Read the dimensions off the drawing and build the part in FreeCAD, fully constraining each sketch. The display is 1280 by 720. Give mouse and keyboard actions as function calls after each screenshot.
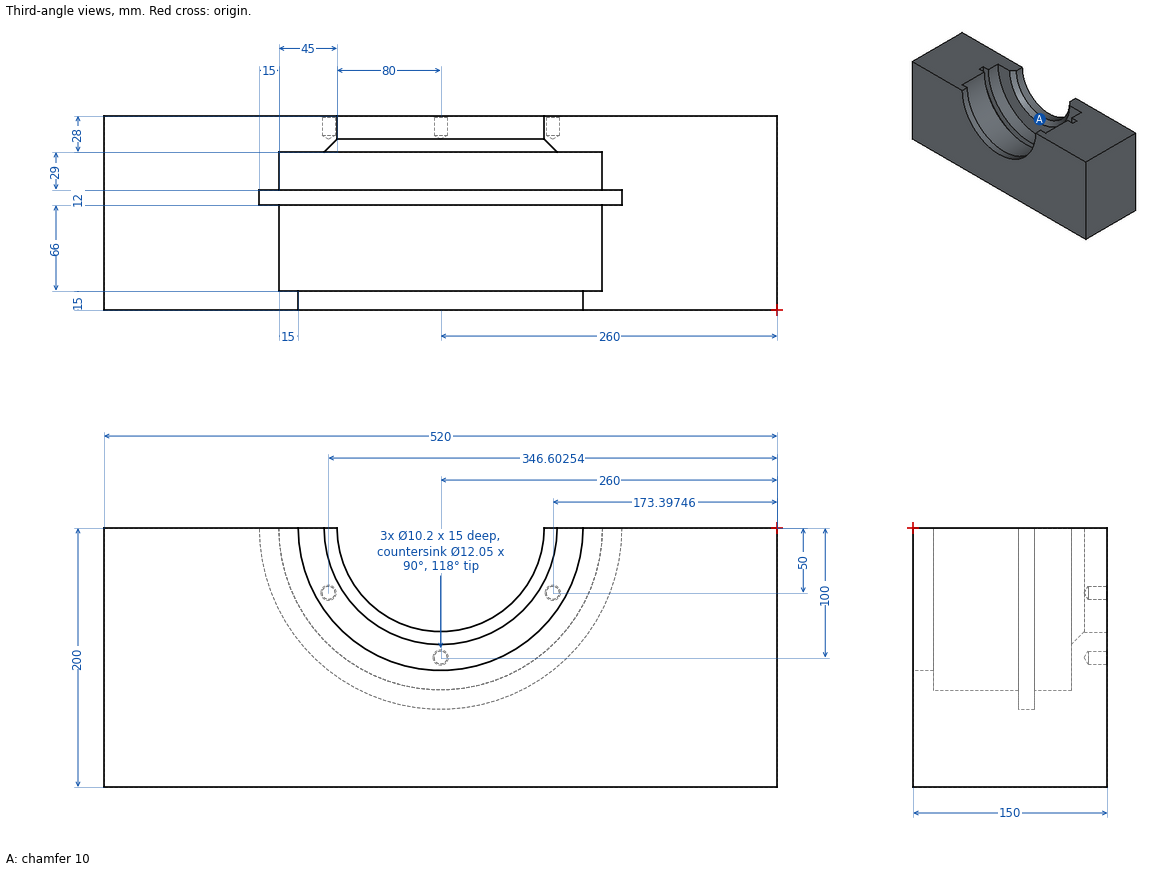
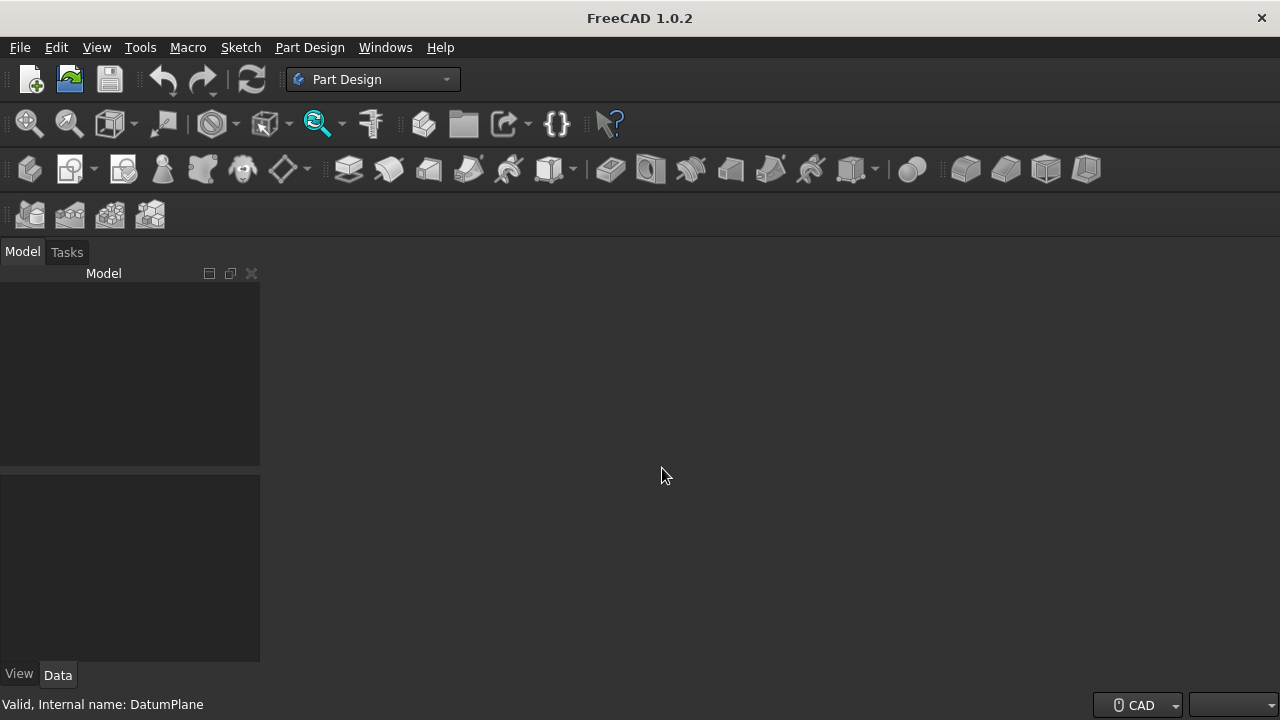
click(30, 80)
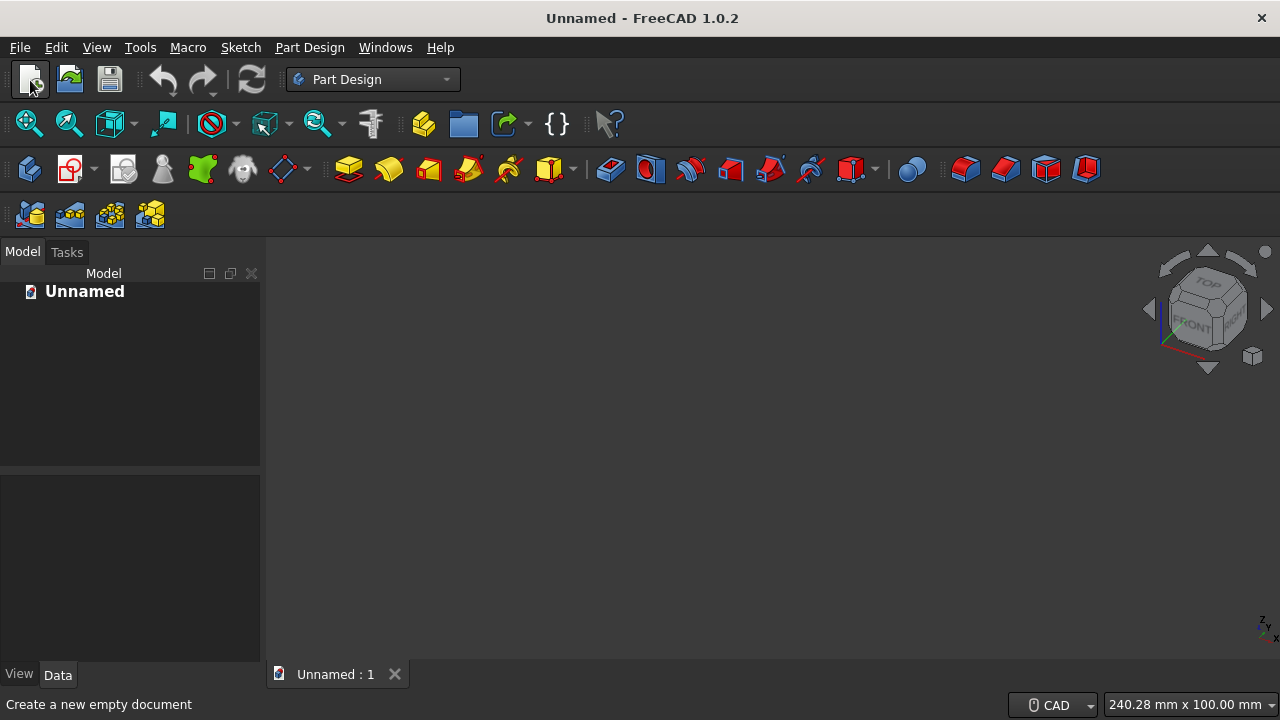
click(70, 170)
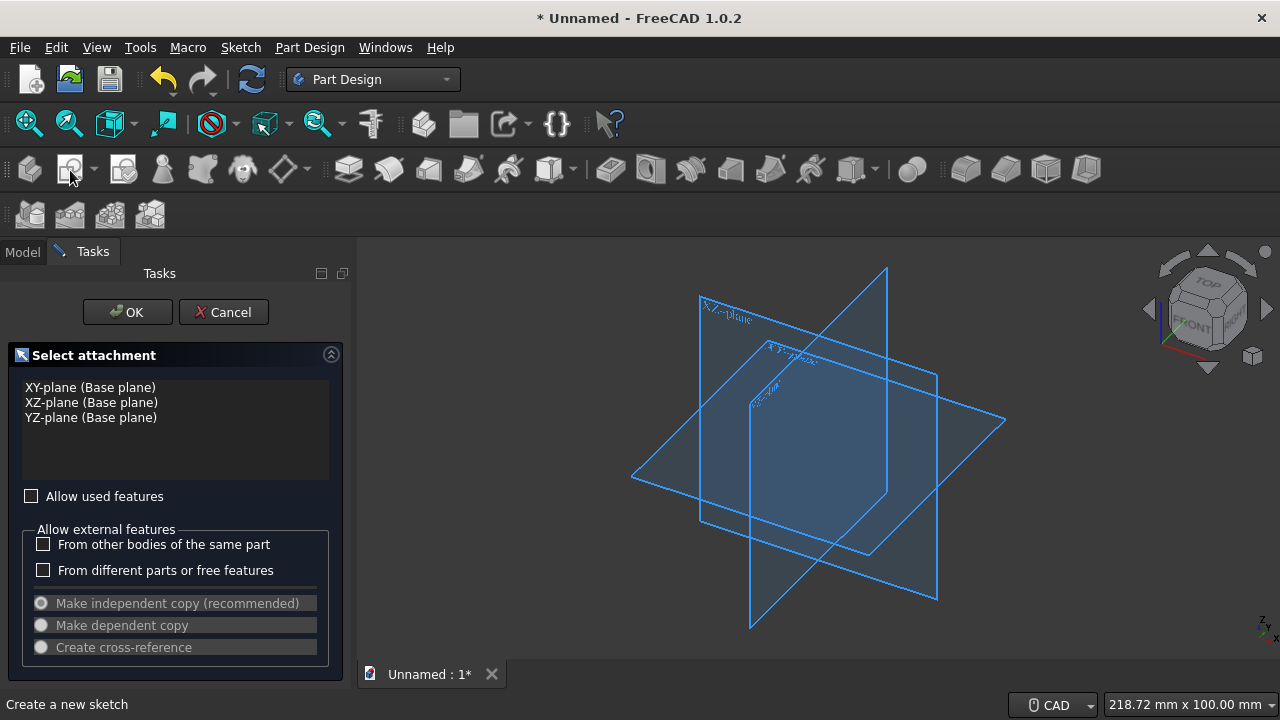
click(82, 402)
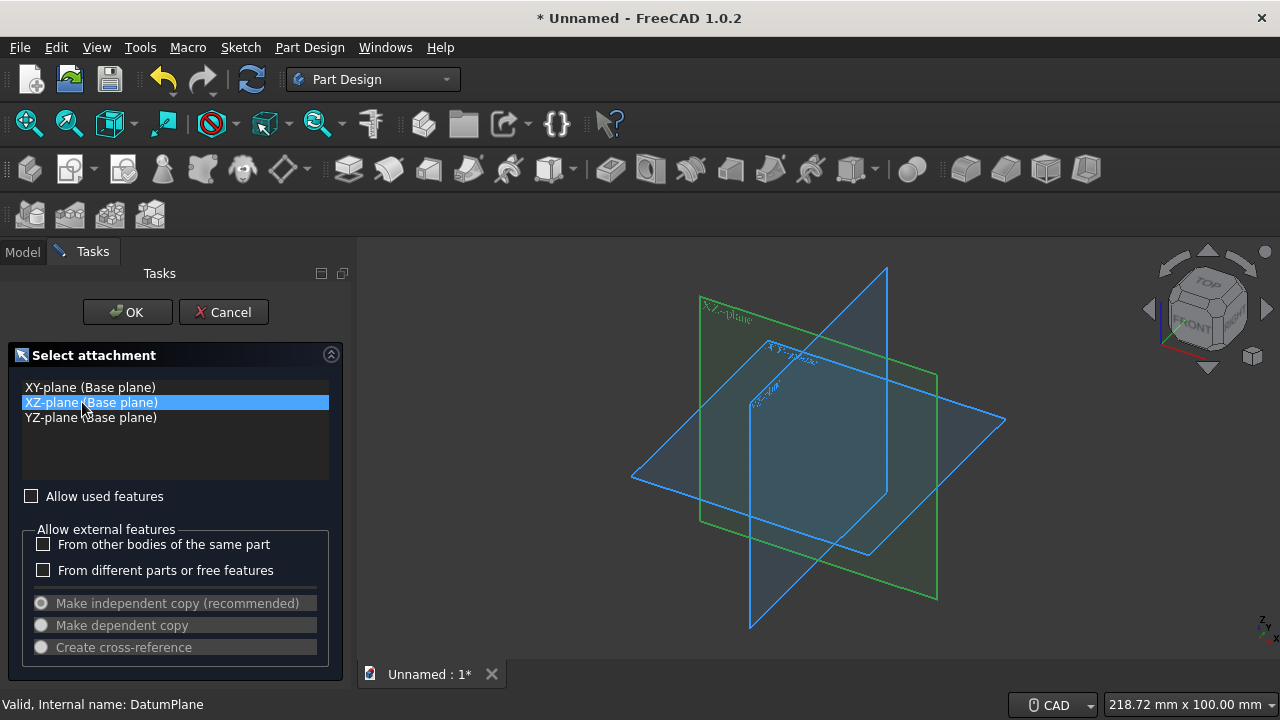
click(128, 312)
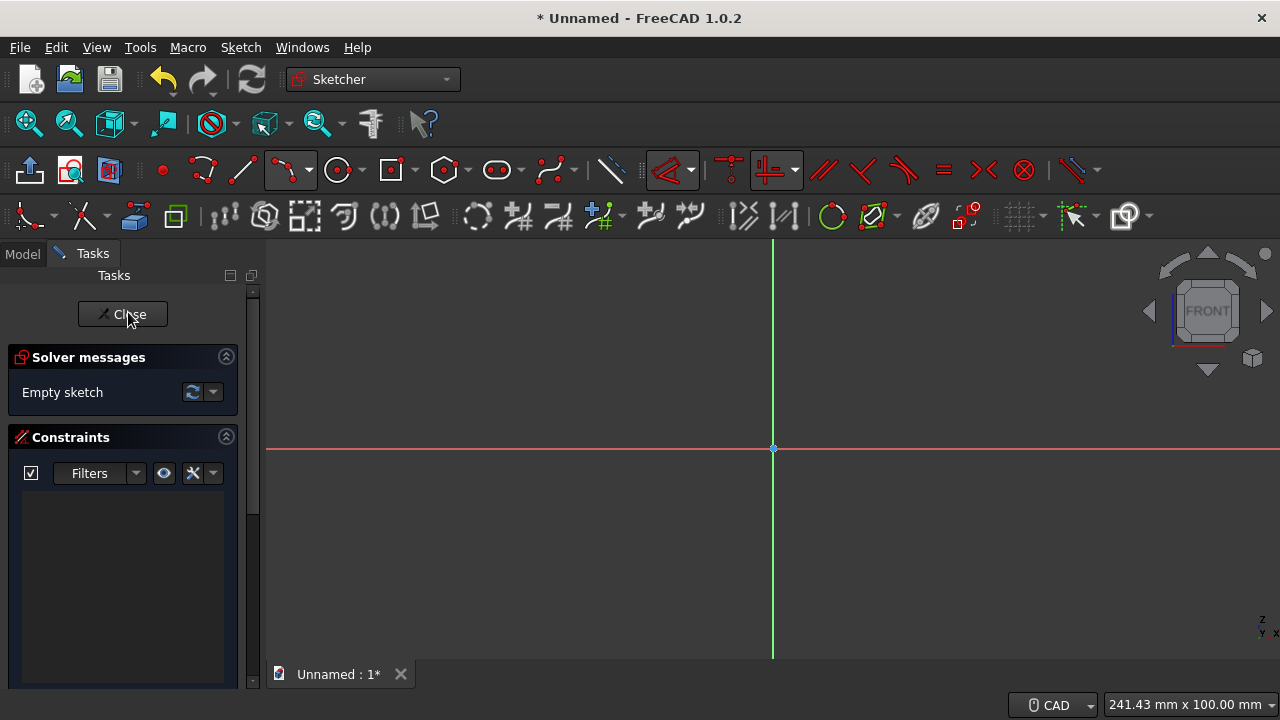
scroll(1040, 312, down, 7)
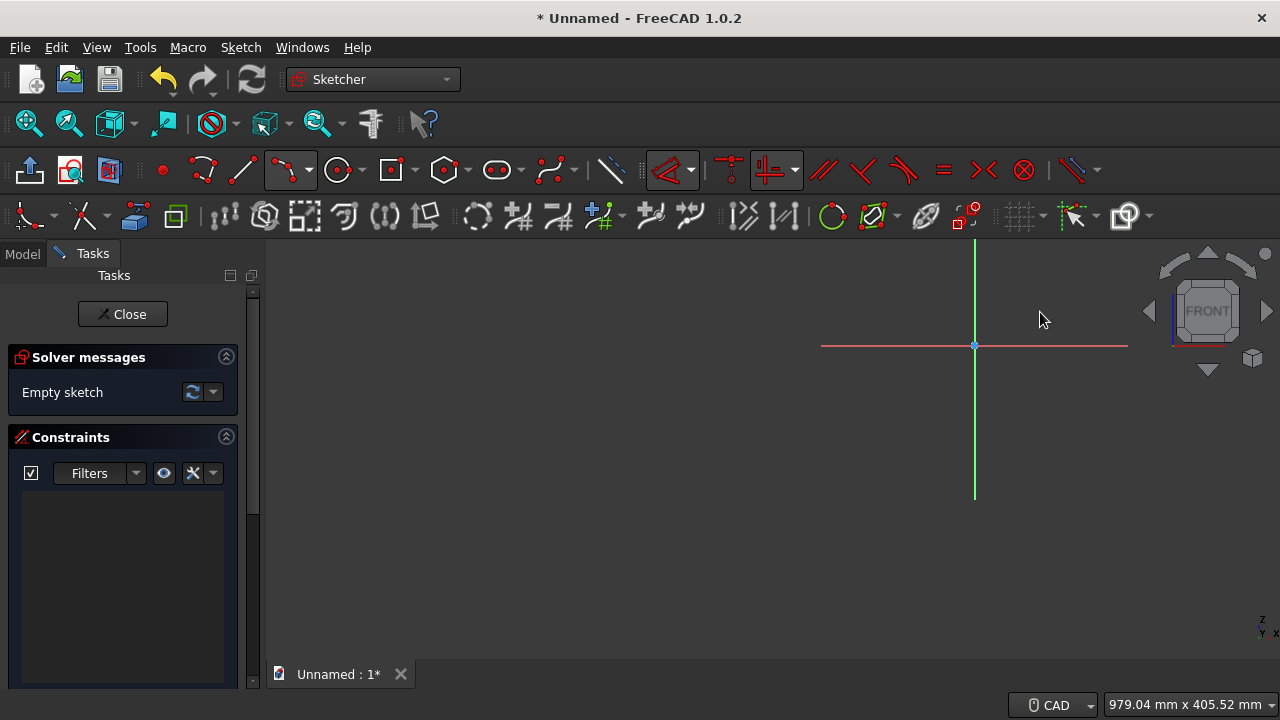
click(418, 170)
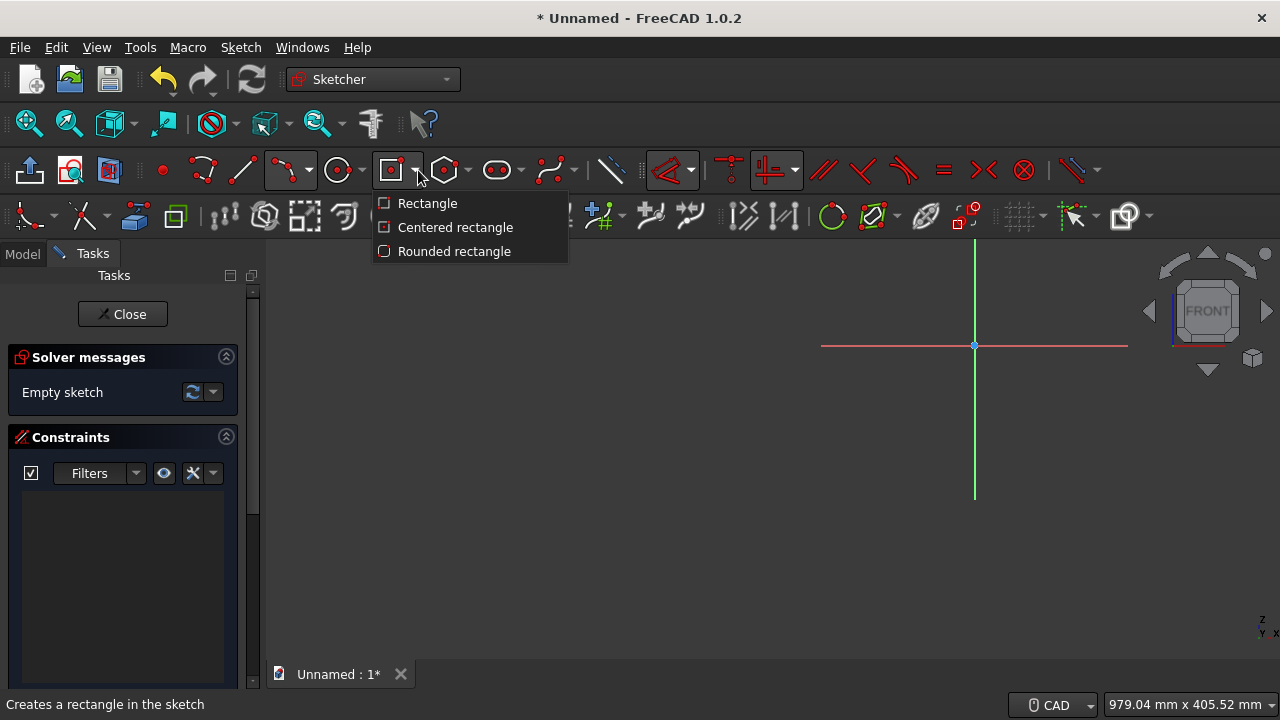
click(470, 203)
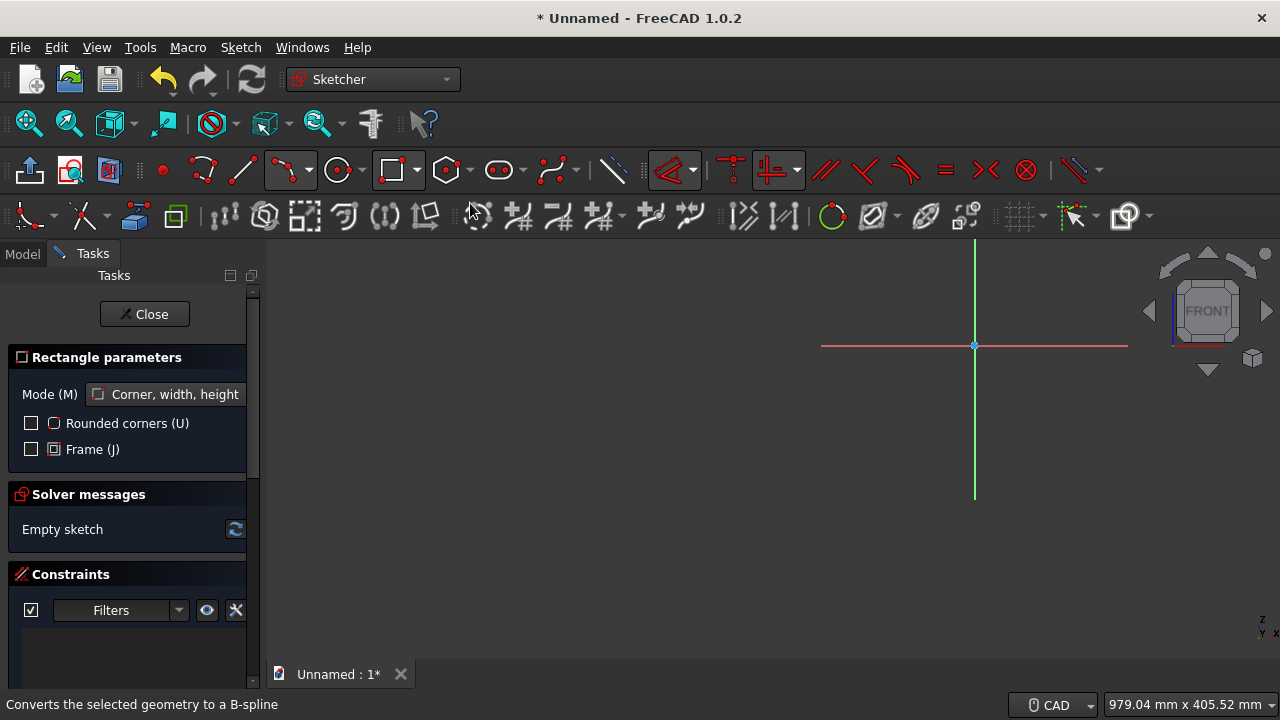
click(975, 346)
click(436, 553)
key(Escape)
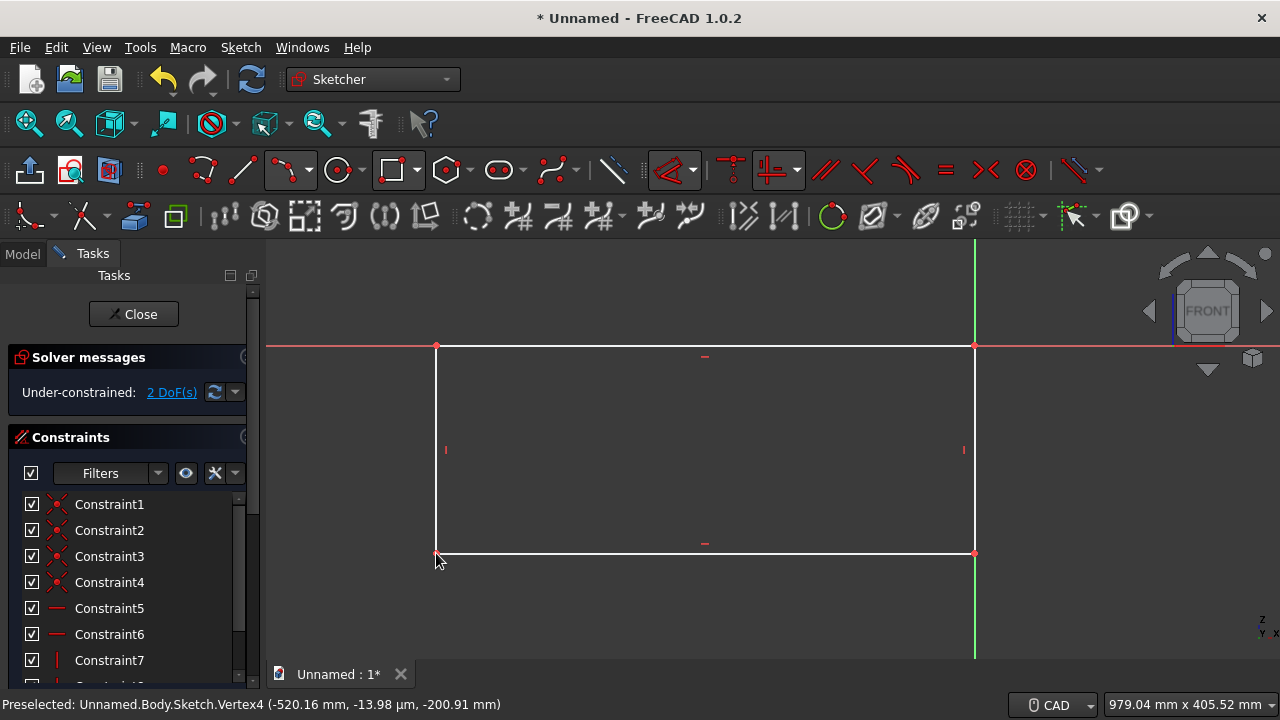
click(668, 170)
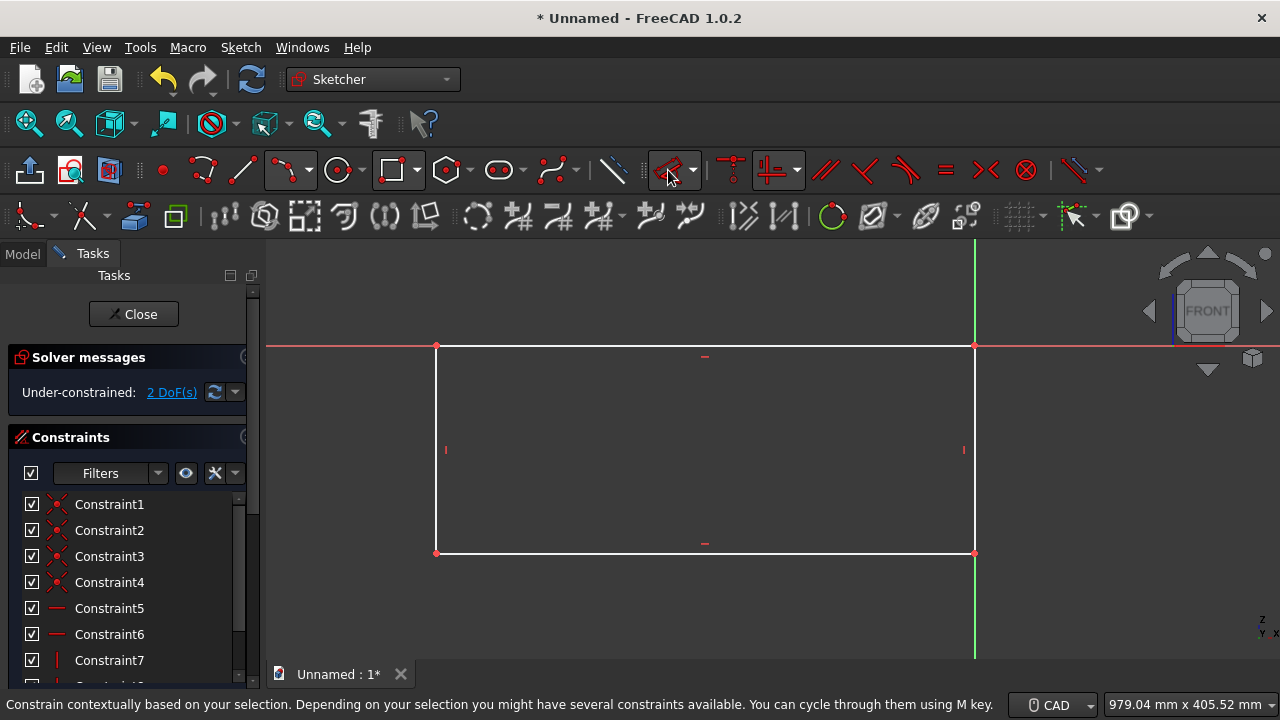
click(813, 346)
click(705, 312)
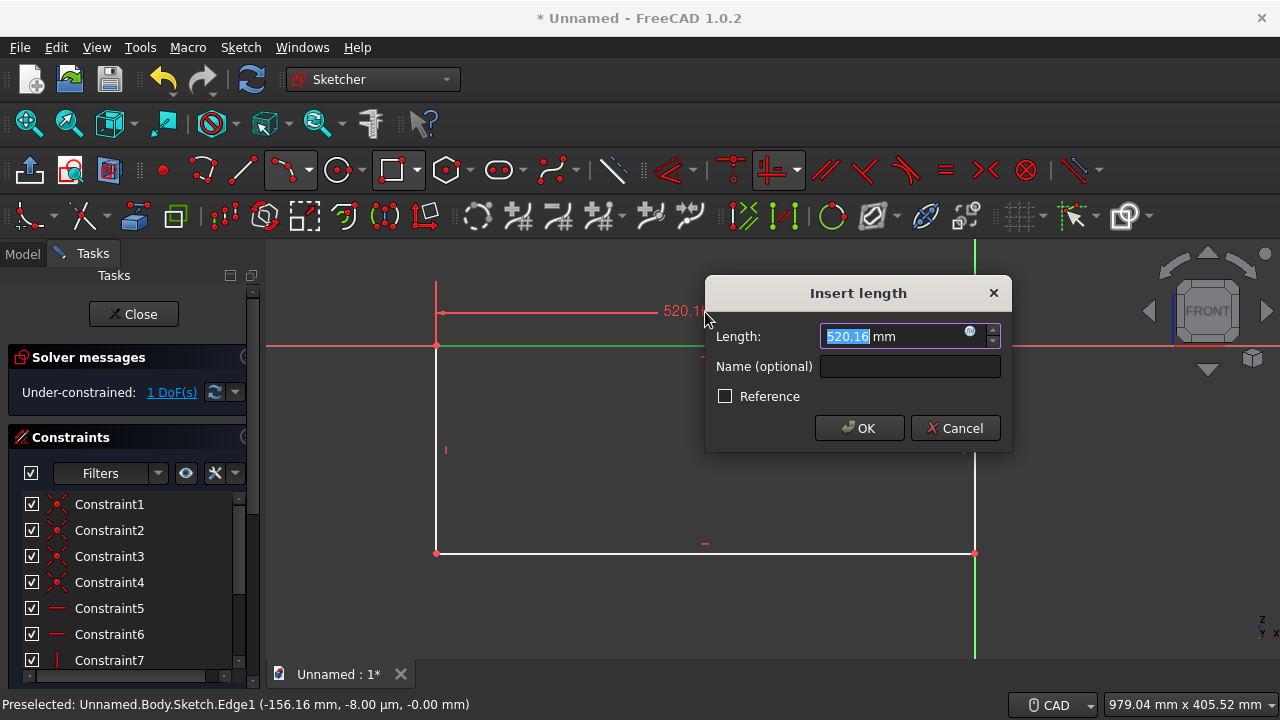
text(520)
key(Return)